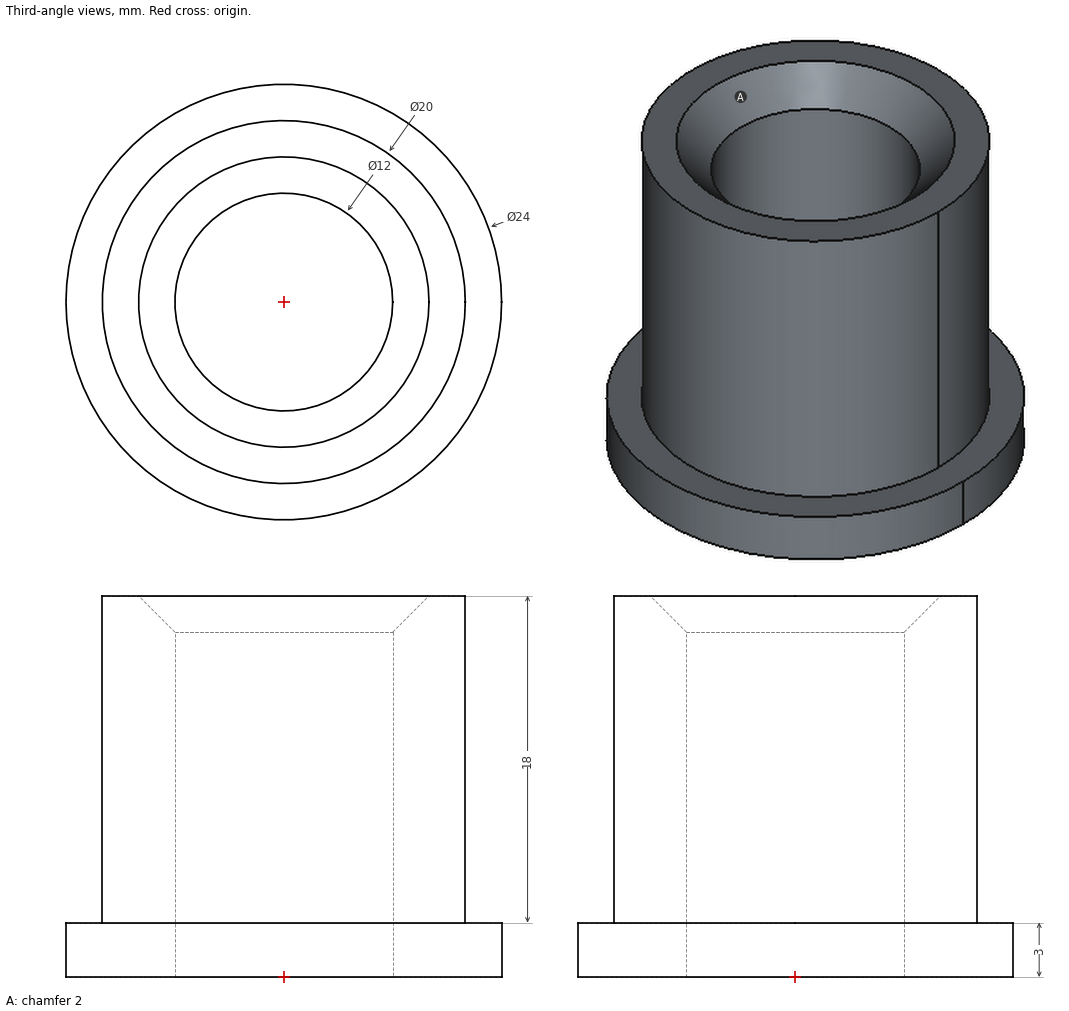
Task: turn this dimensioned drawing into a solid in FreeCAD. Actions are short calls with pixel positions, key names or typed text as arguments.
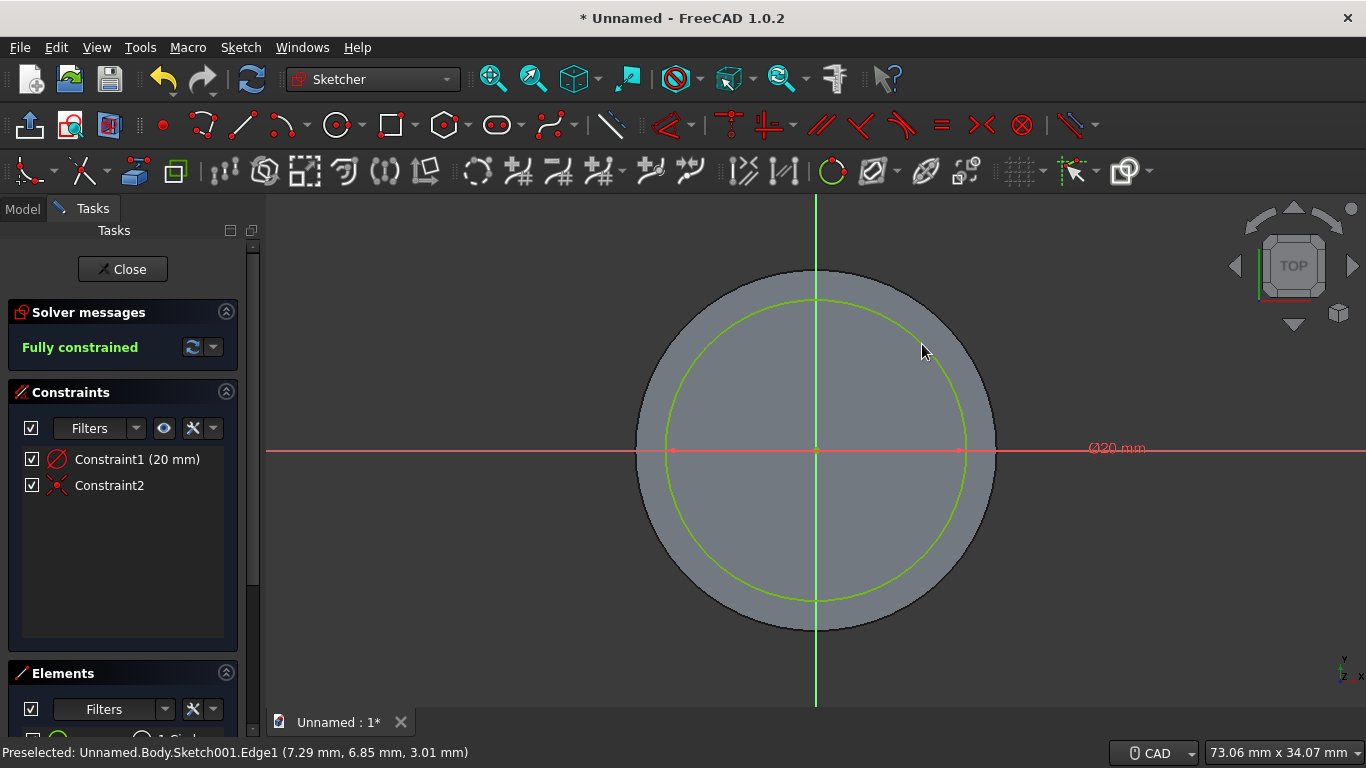
click(123, 269)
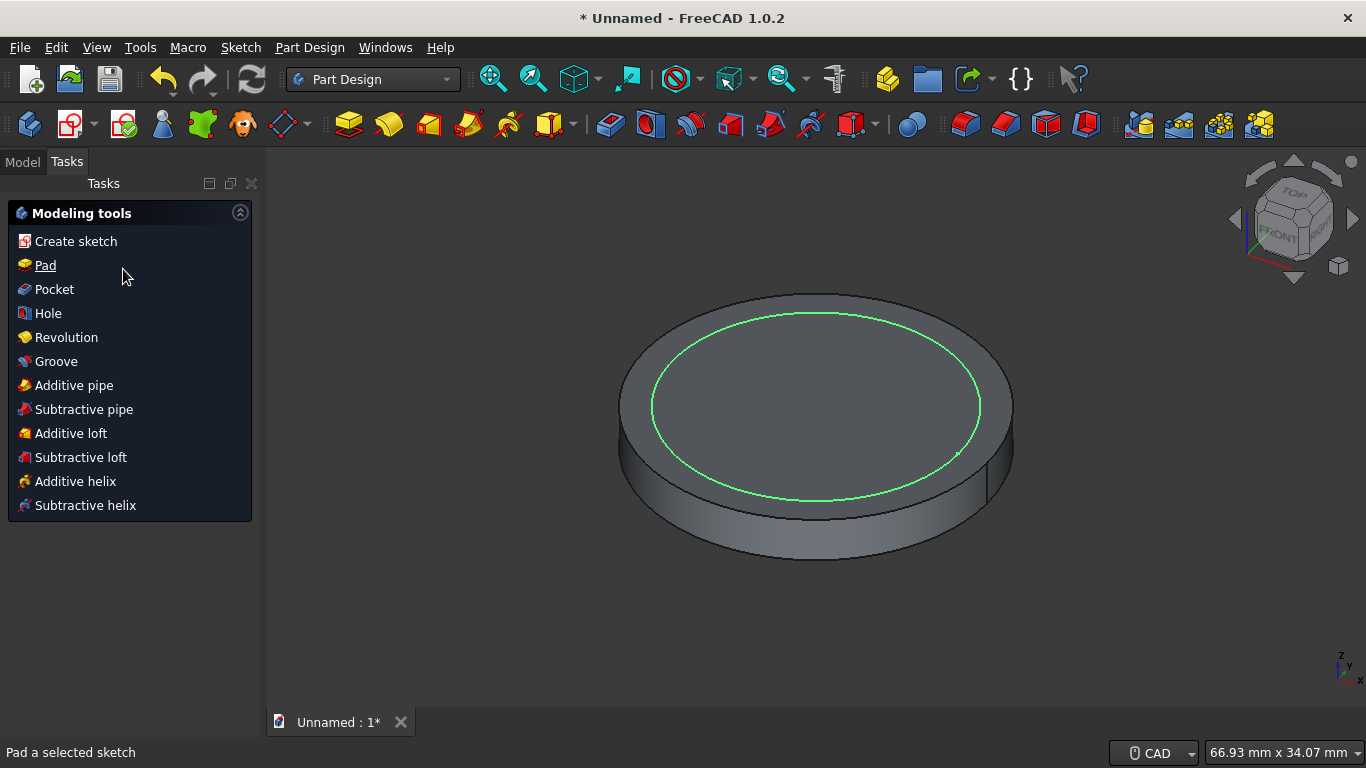
click(350, 124)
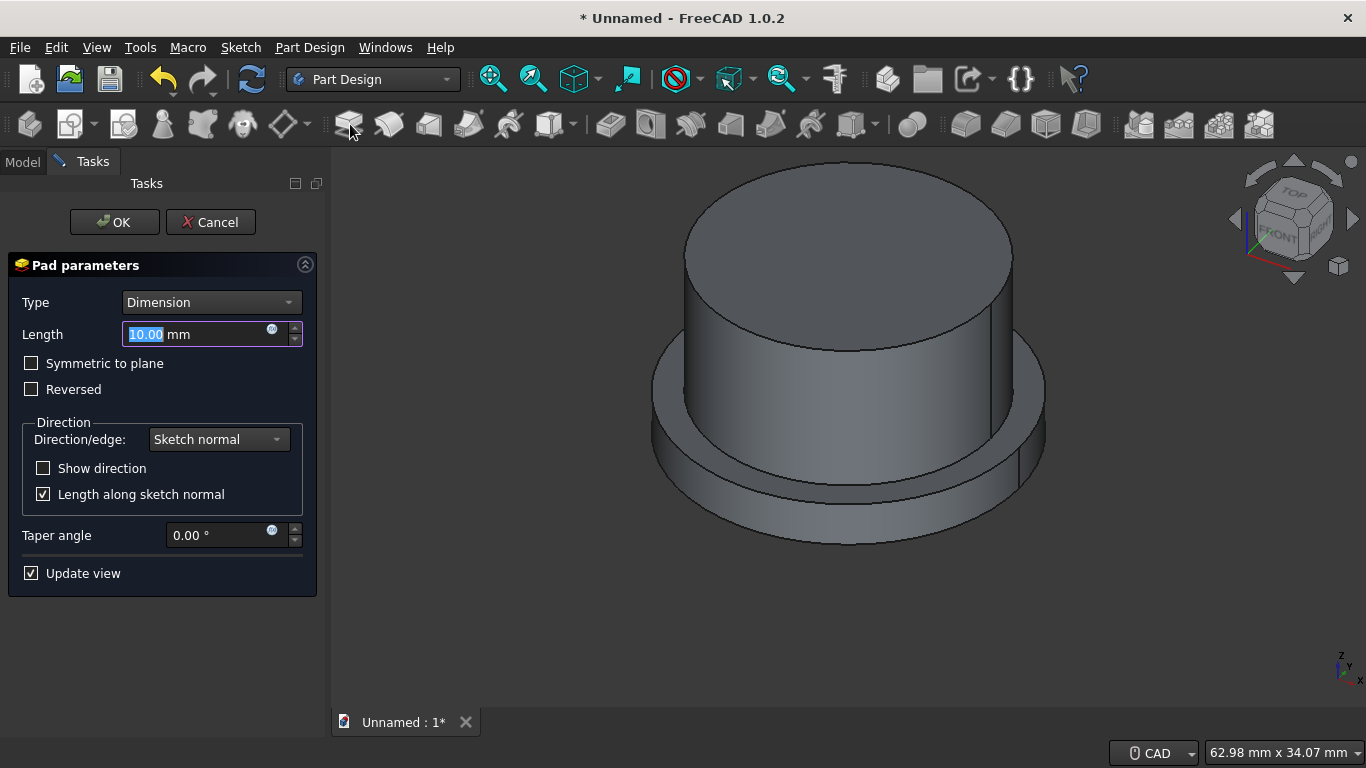
text(18)
key(Tab)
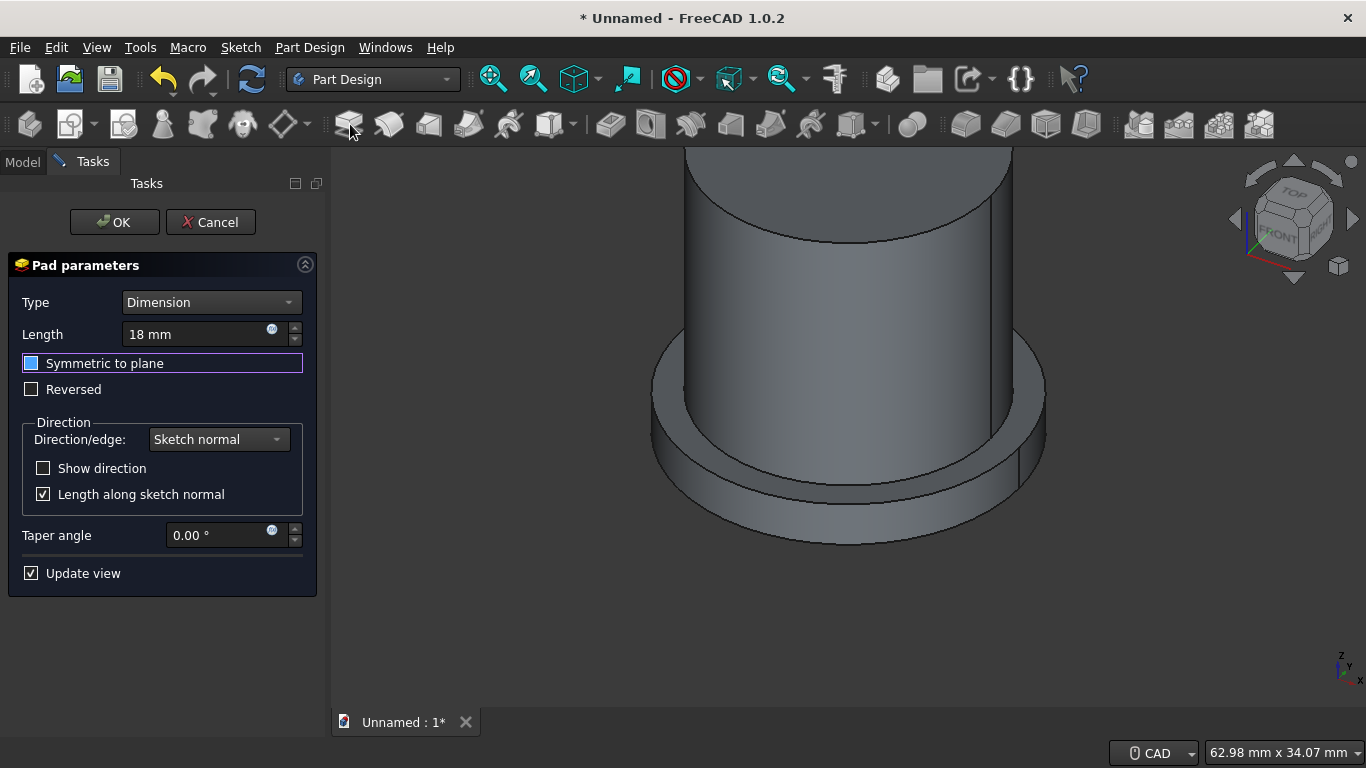
click(115, 222)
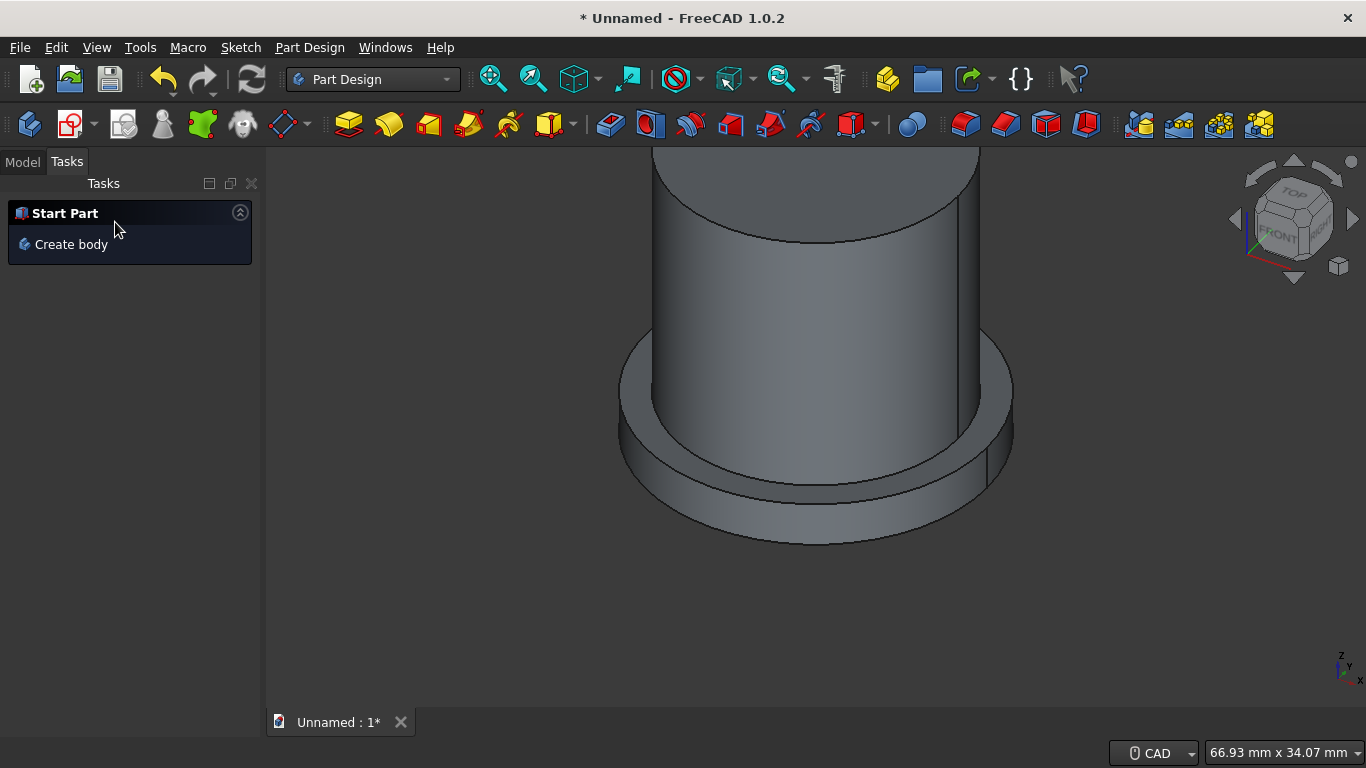
click(494, 80)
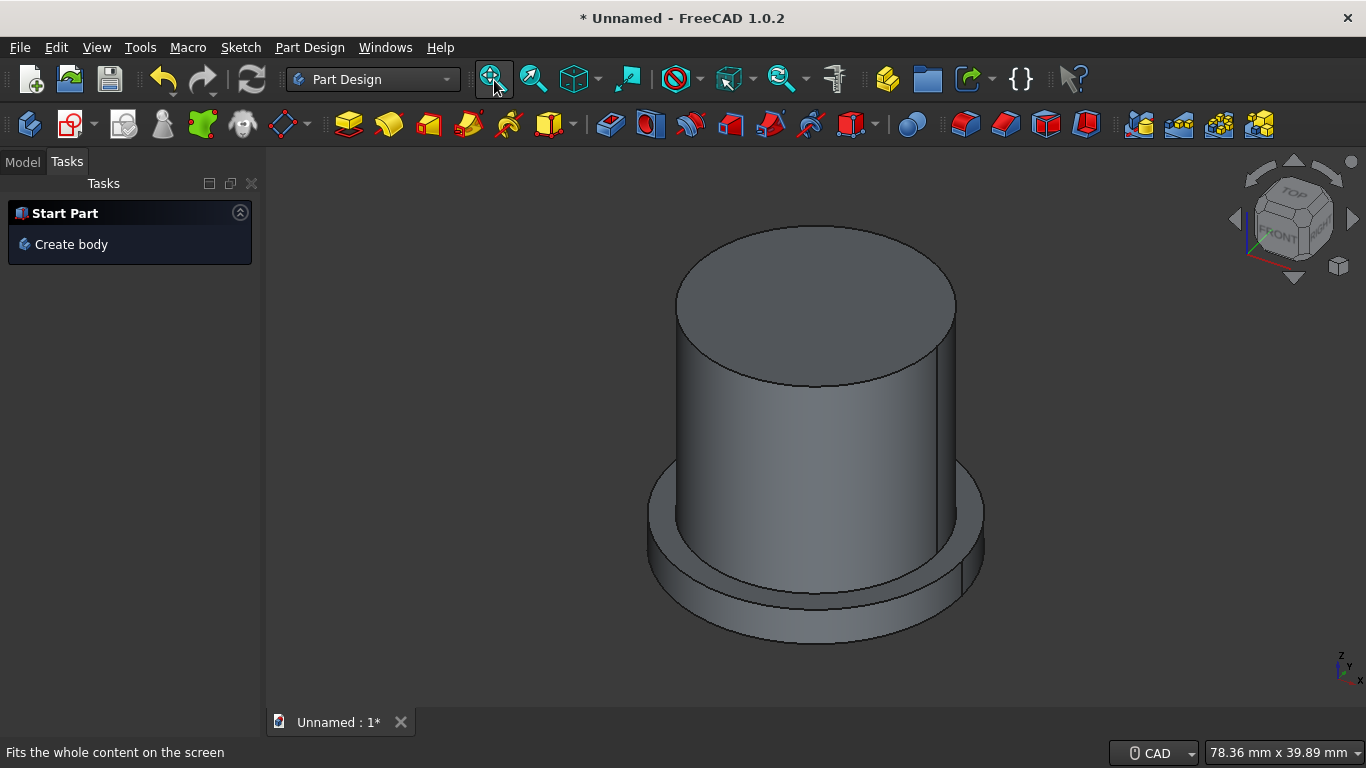
click(816, 305)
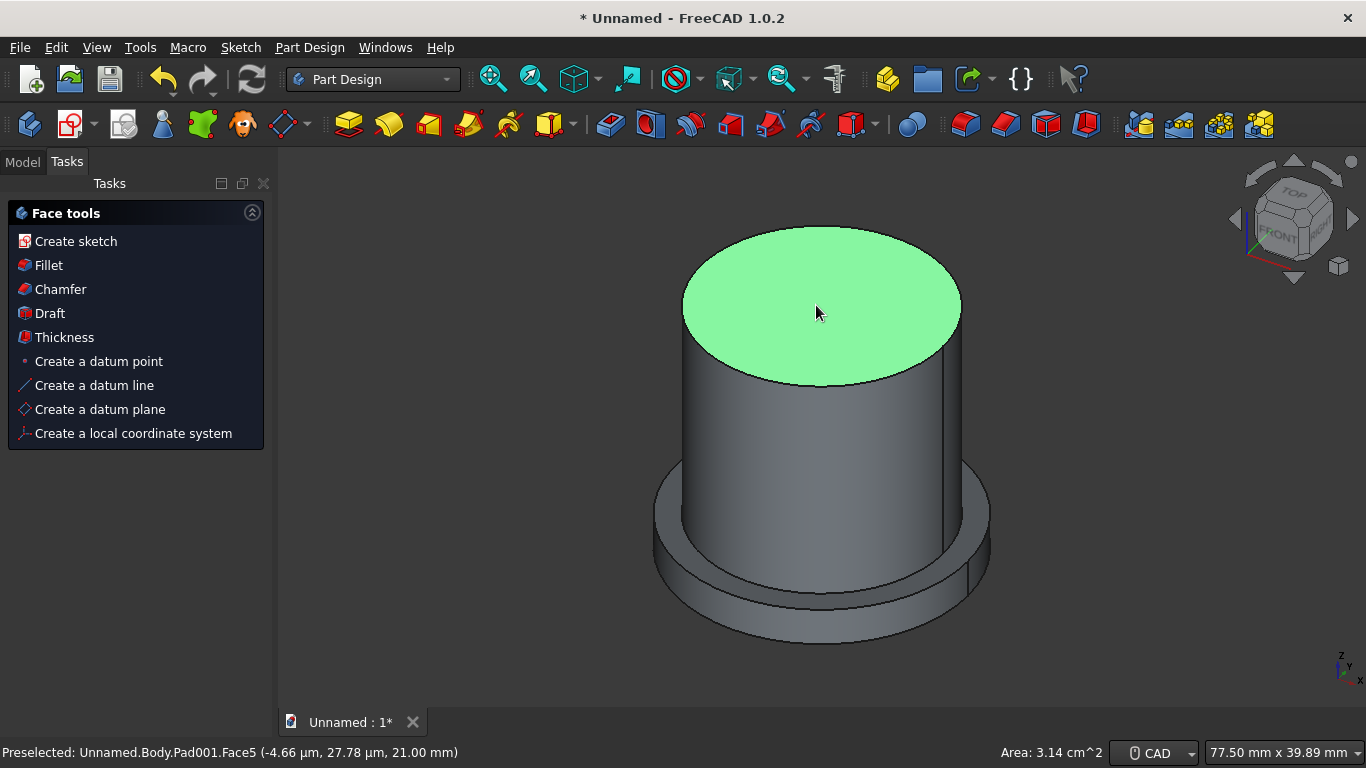
click(70, 124)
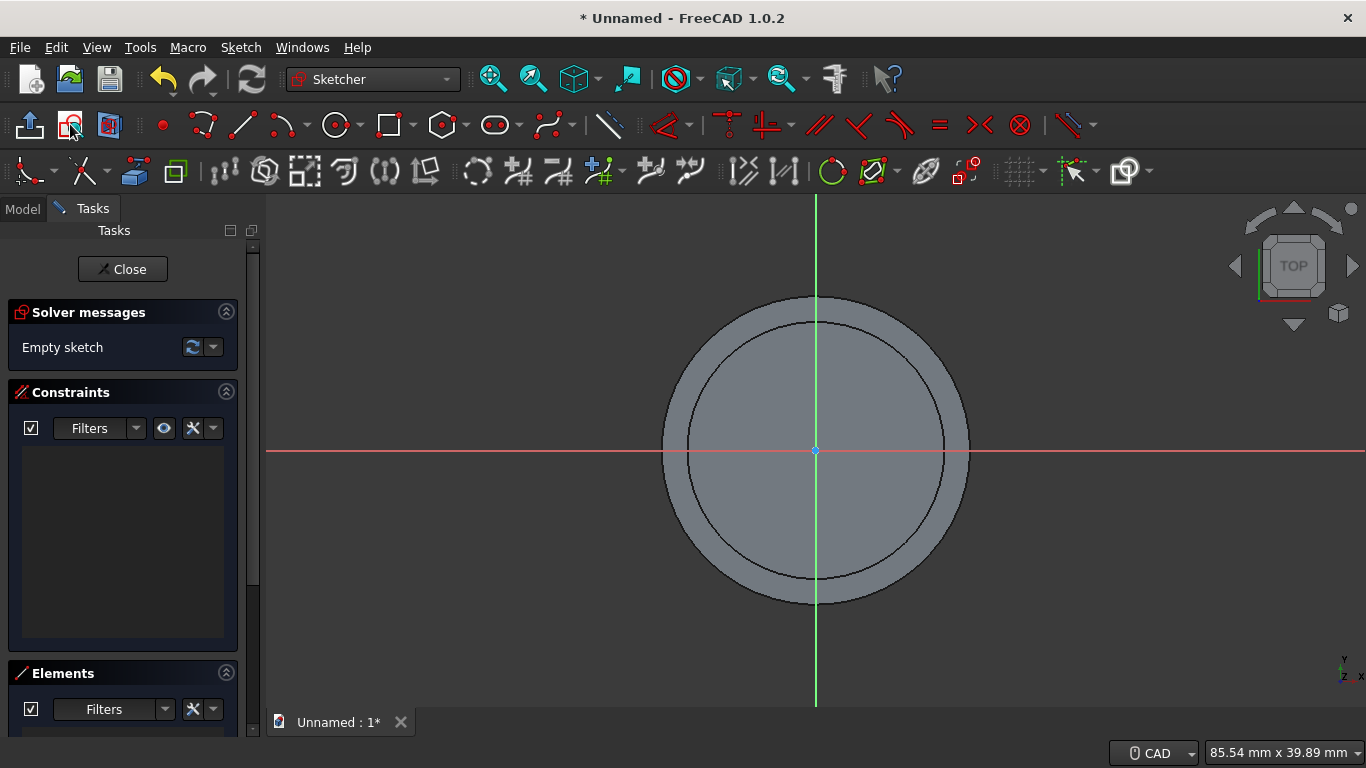
scroll(872, 450, up, 4)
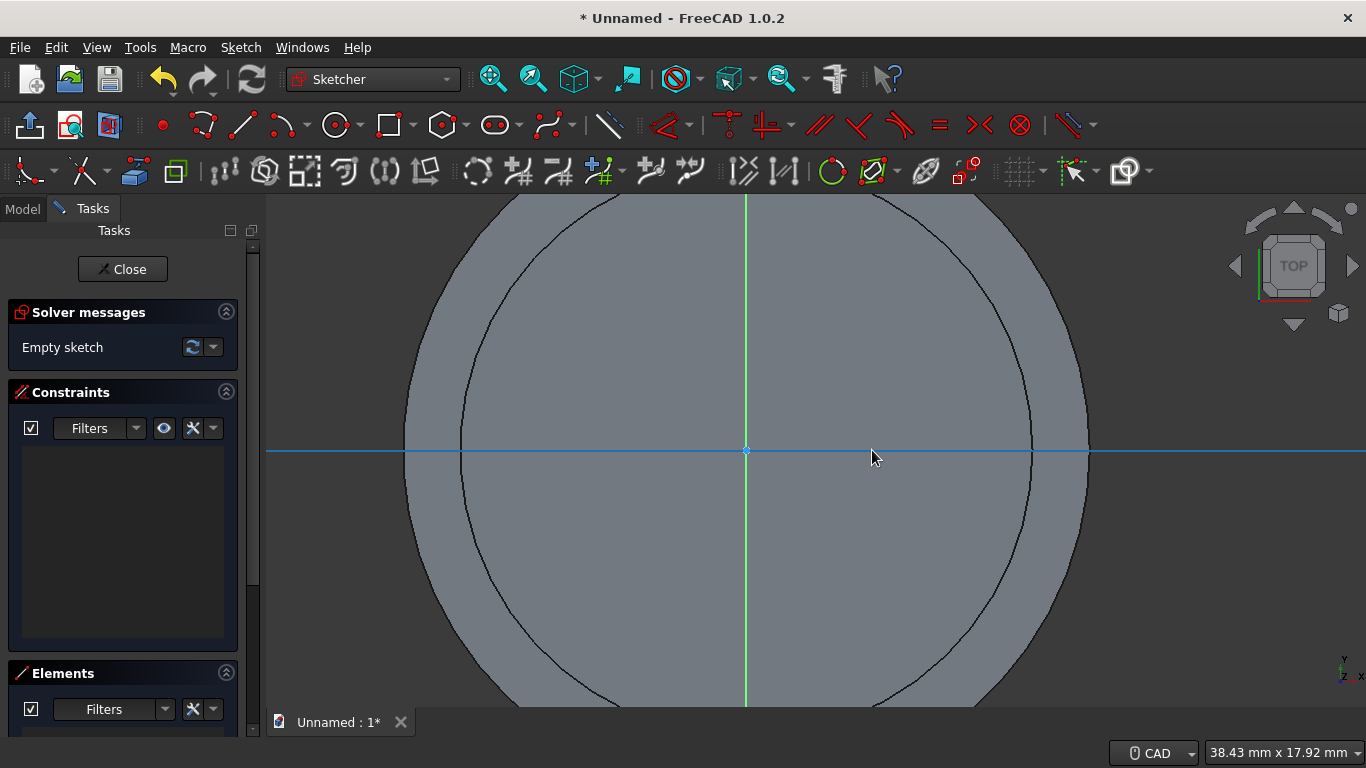
click(336, 126)